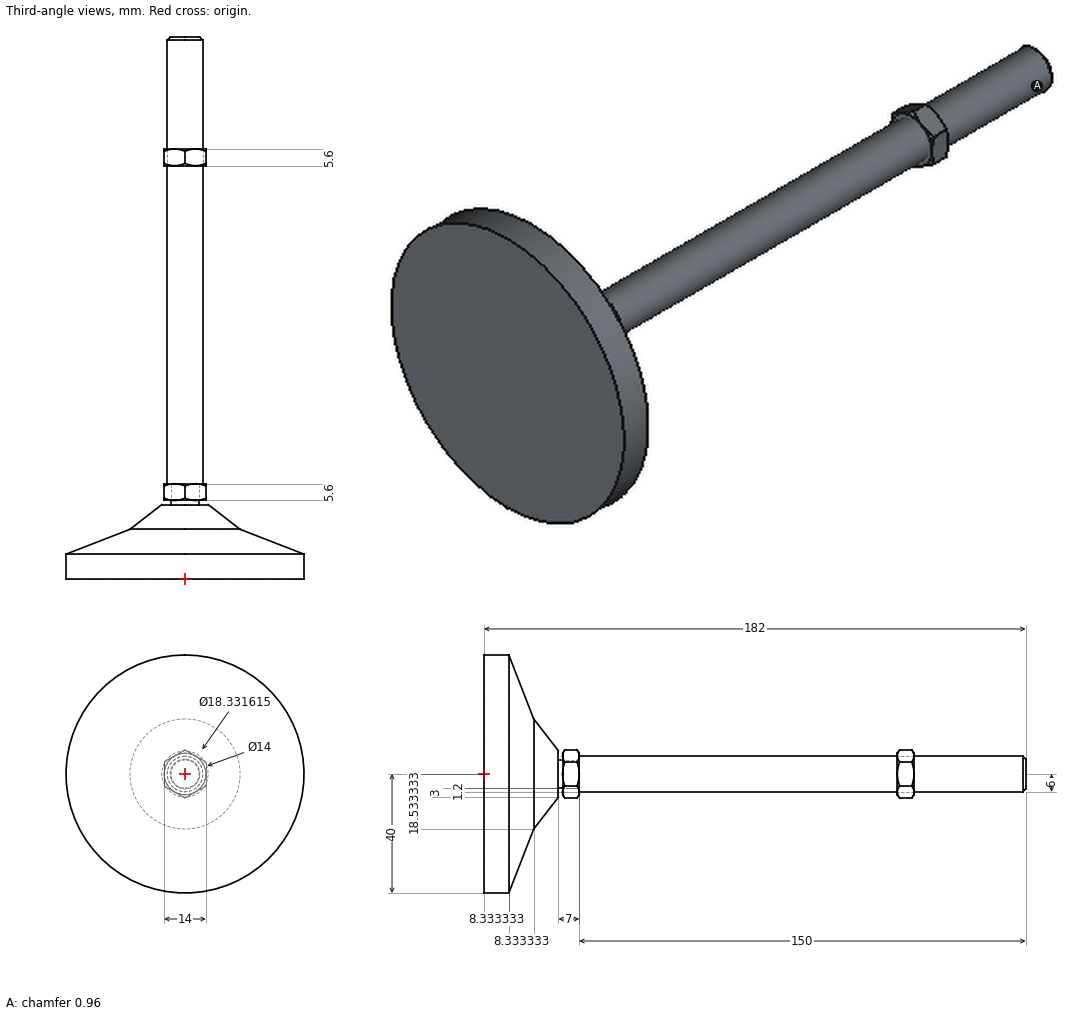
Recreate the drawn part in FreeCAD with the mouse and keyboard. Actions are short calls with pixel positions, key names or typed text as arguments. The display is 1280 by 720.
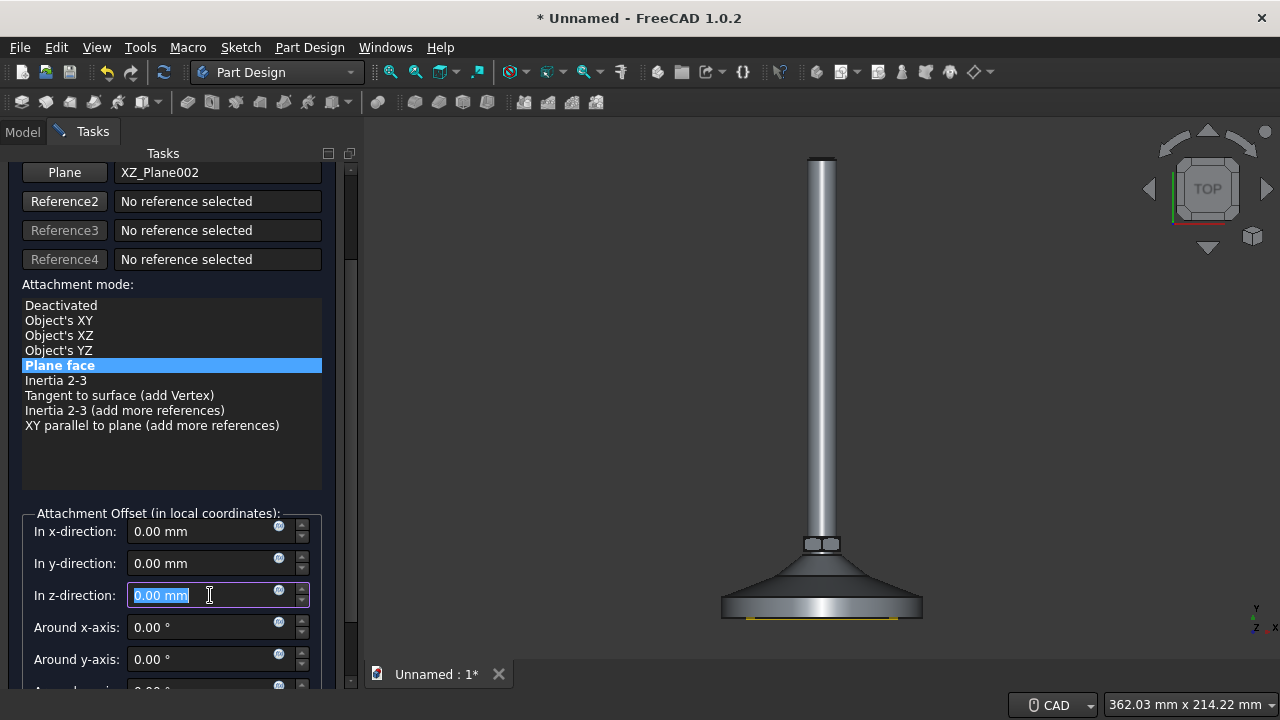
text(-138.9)
key(Tab)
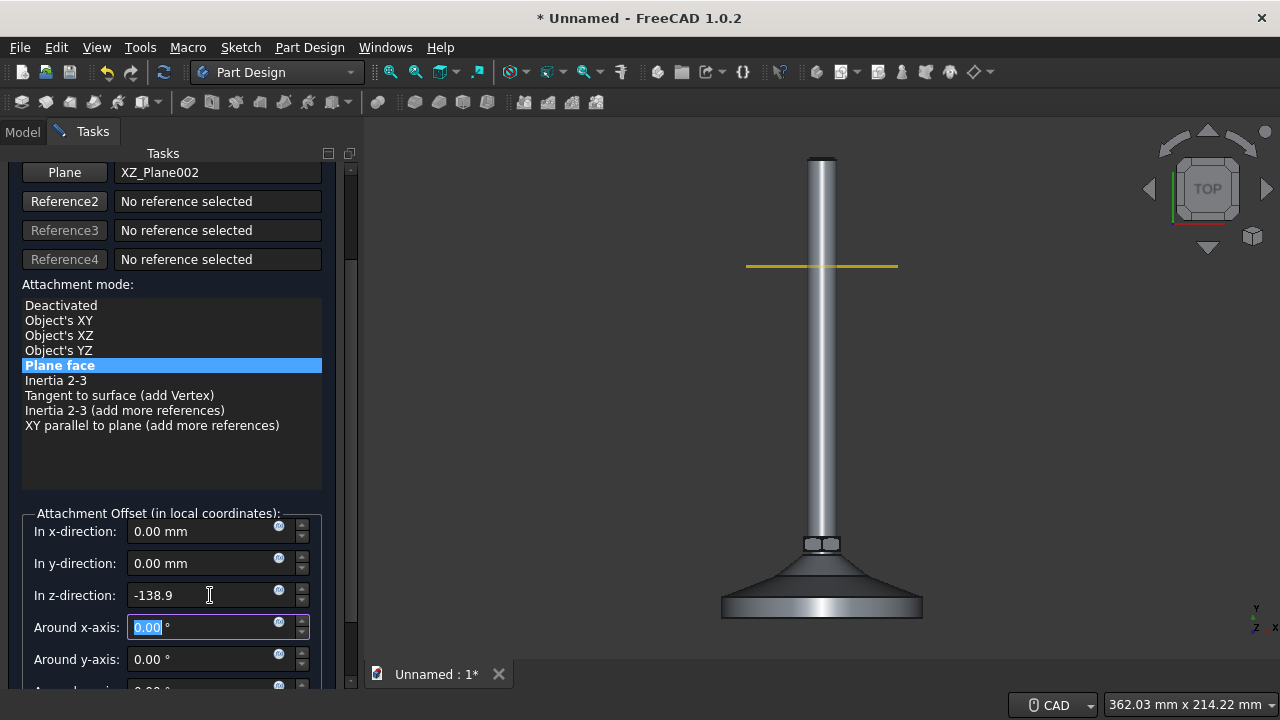
scroll(351, 426, up, 3)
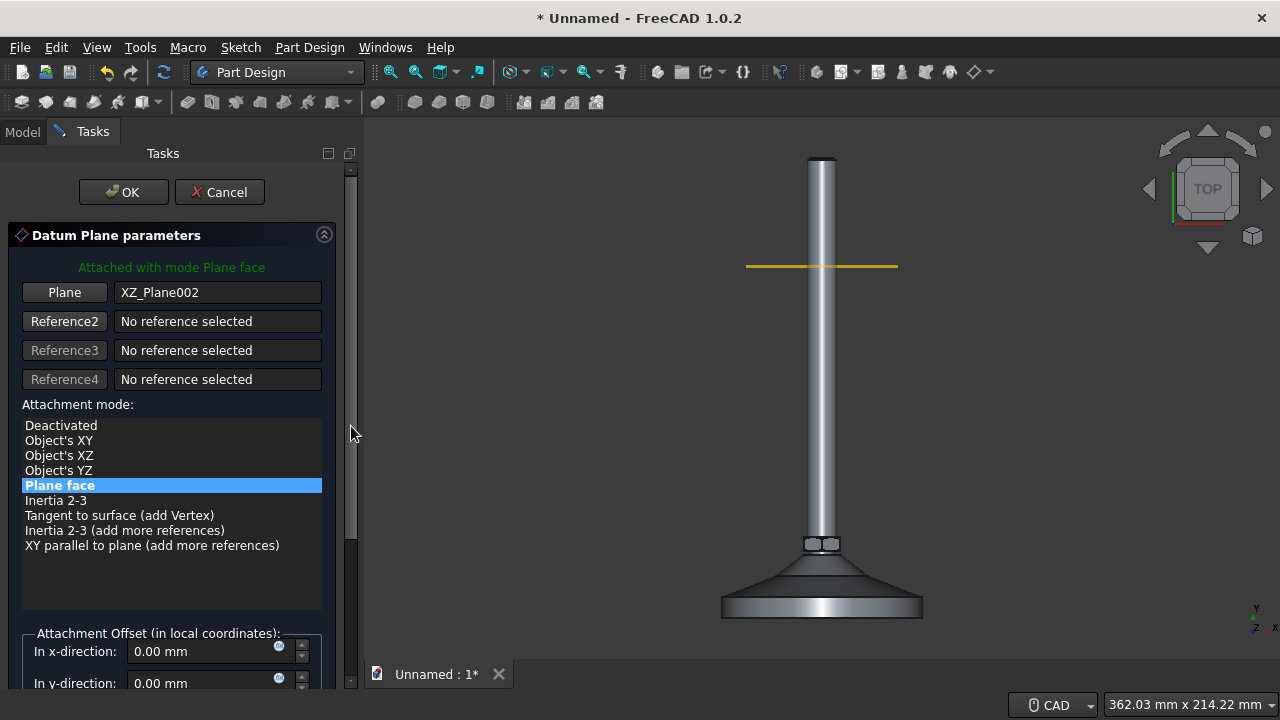
click(124, 192)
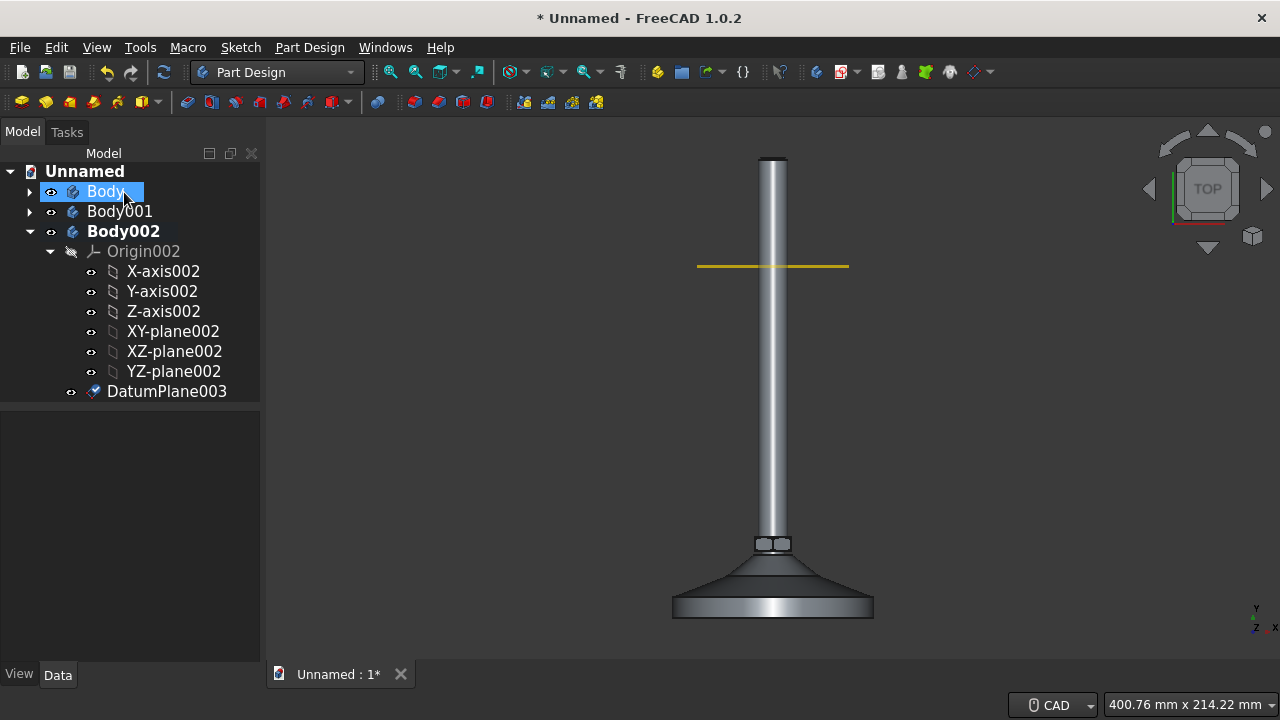
click(116, 392)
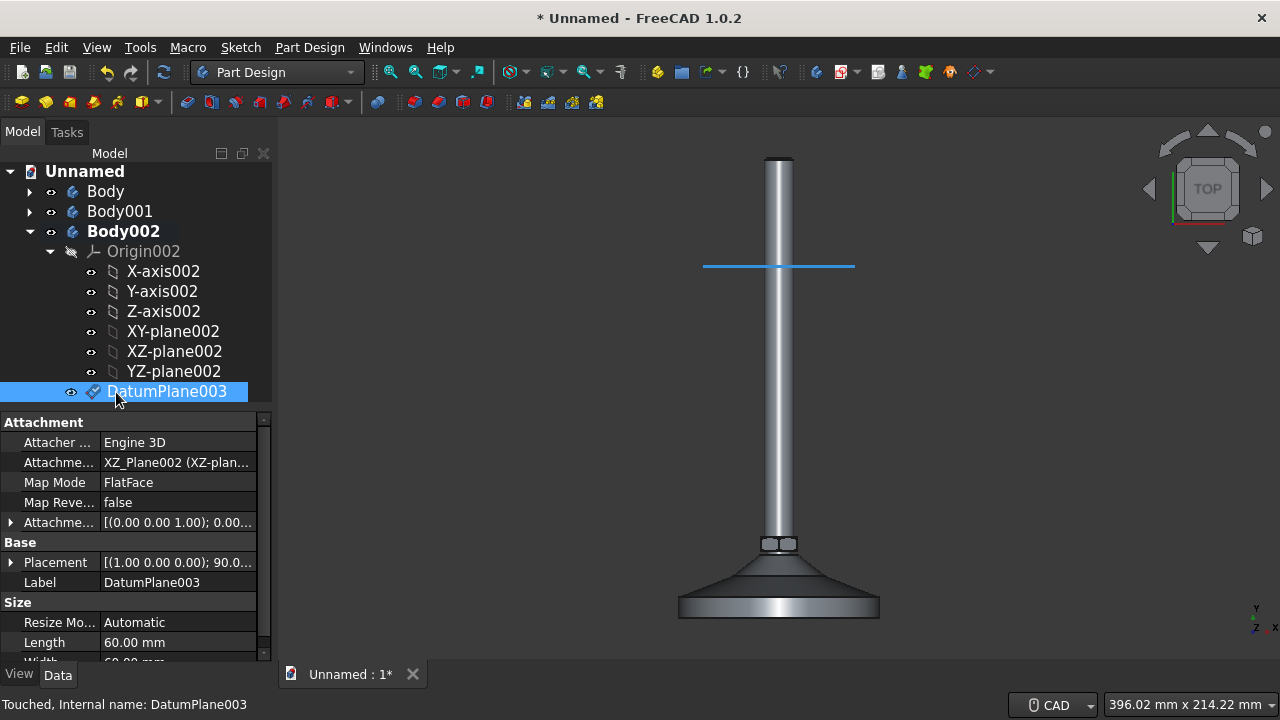
click(842, 72)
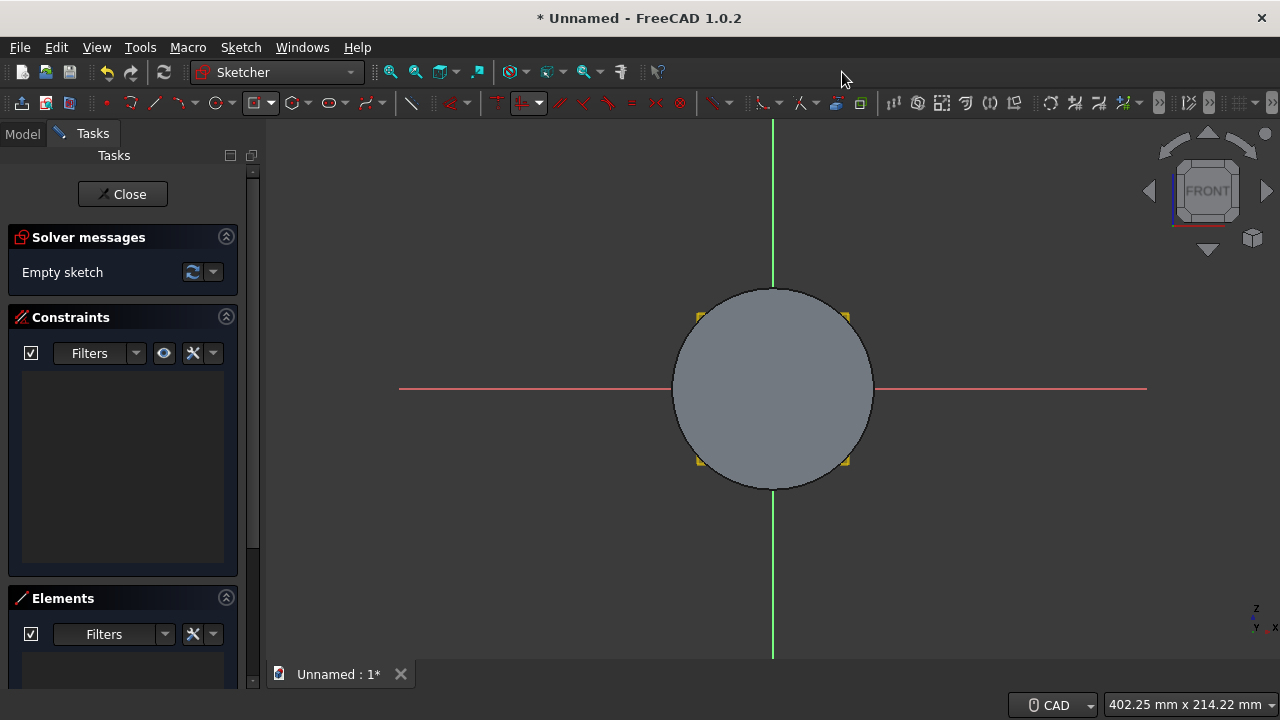
scroll(782, 389, up, 11)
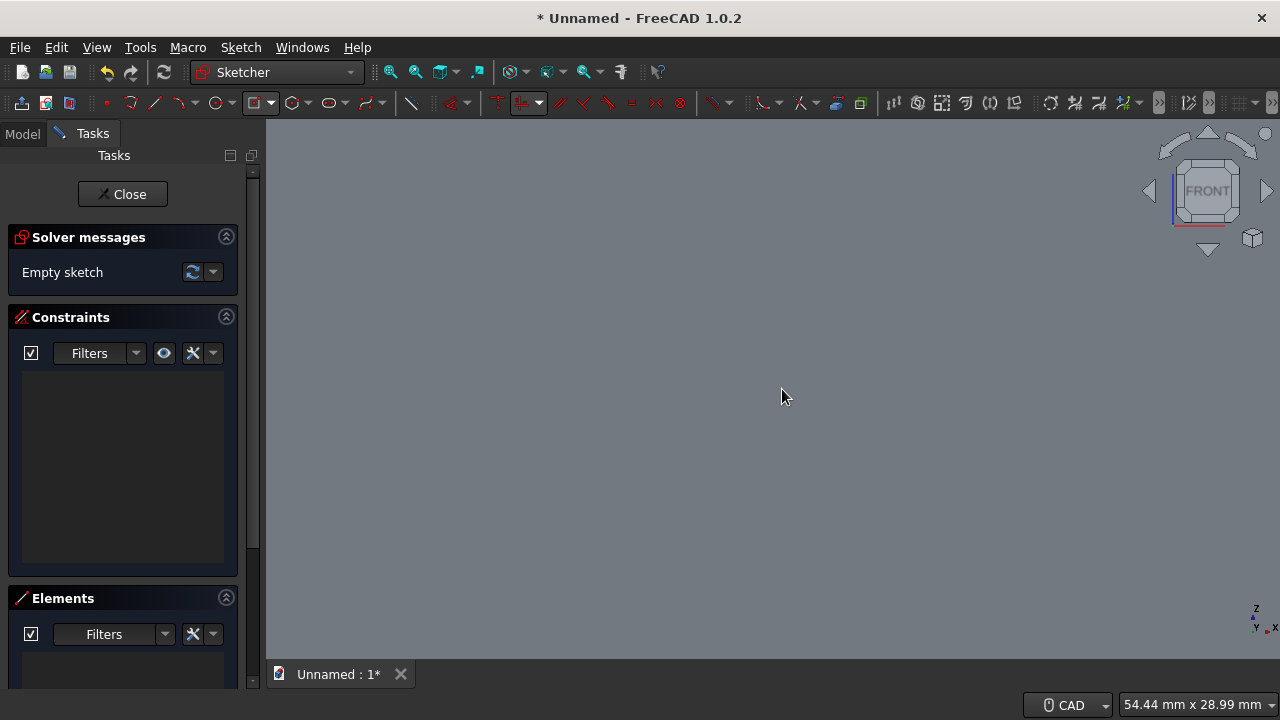
click(292, 104)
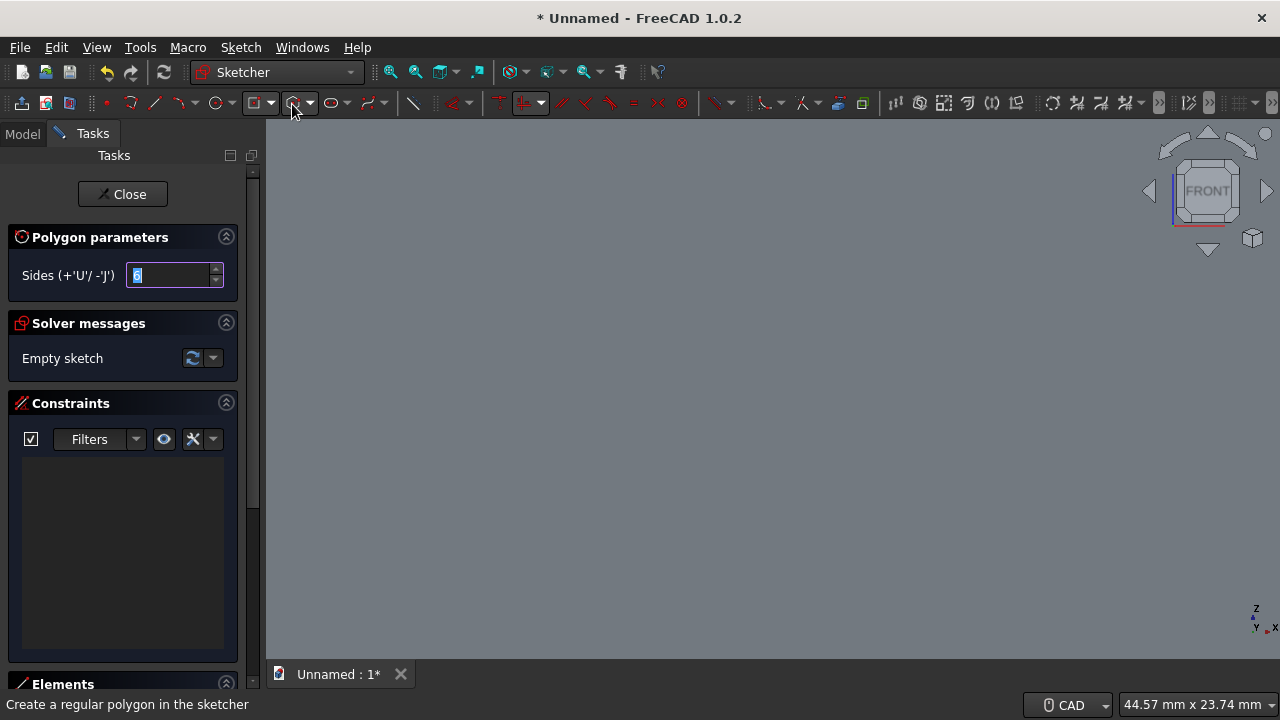
click(697, 385)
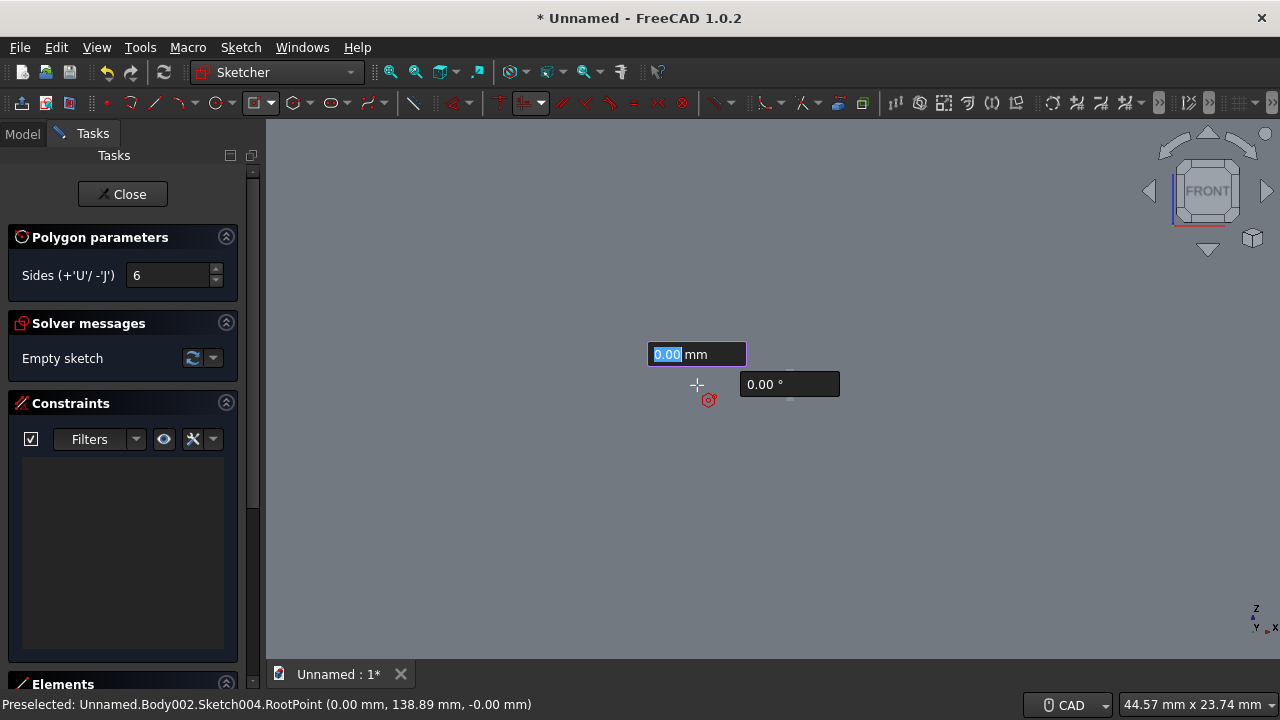
click(697, 569)
right_click(697, 569)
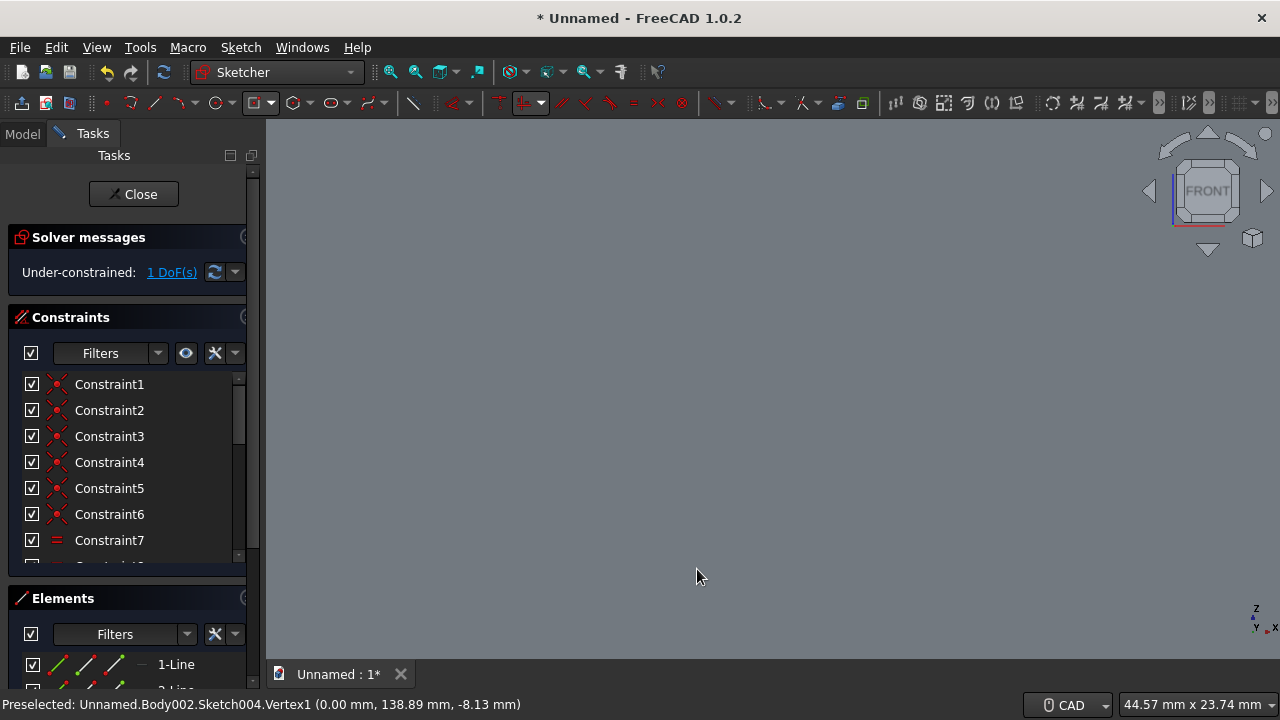
click(452, 104)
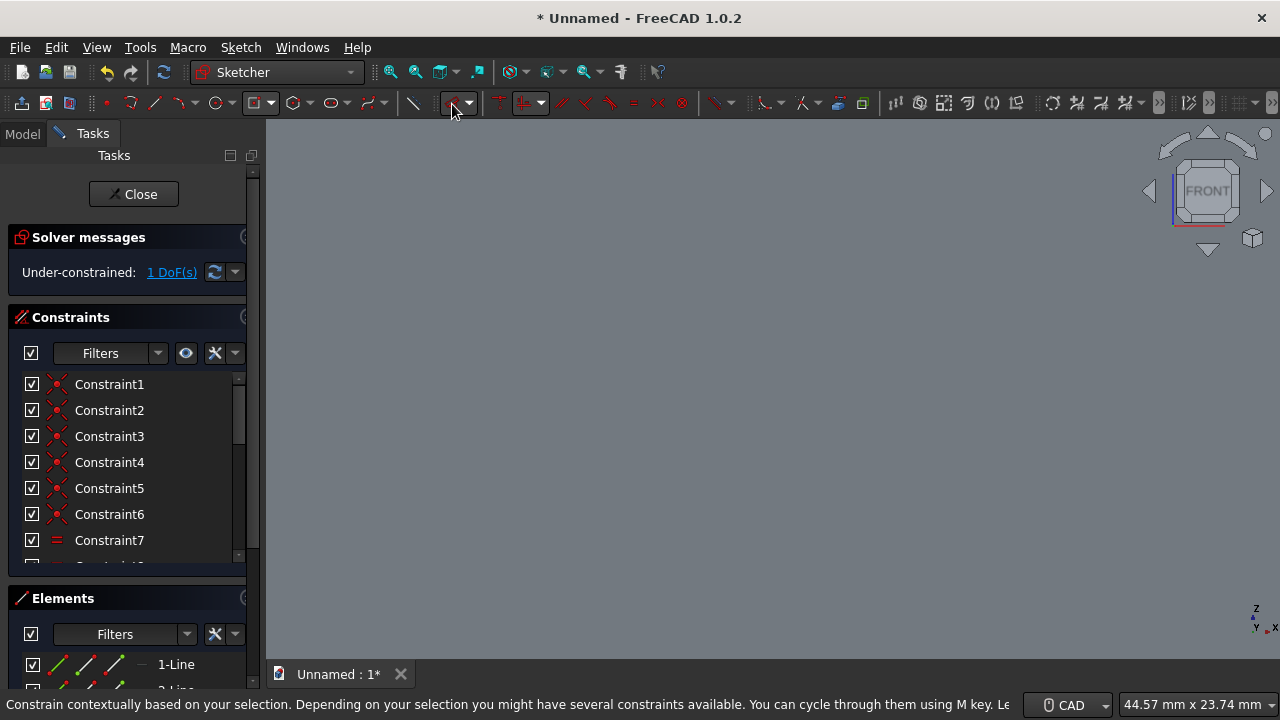
click(536, 292)